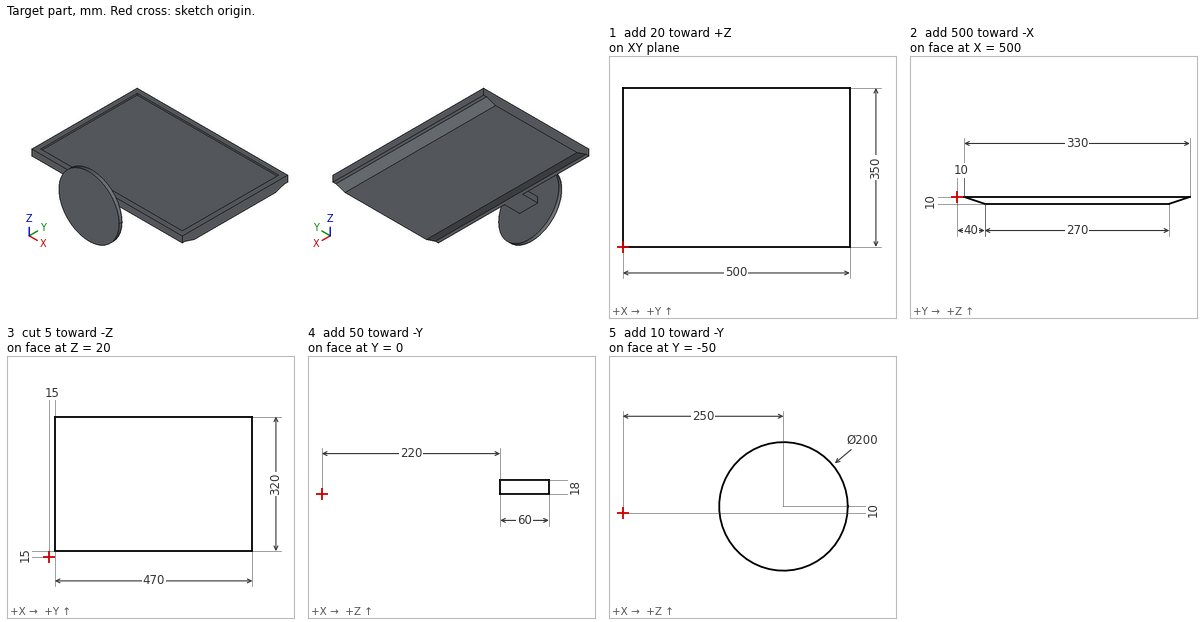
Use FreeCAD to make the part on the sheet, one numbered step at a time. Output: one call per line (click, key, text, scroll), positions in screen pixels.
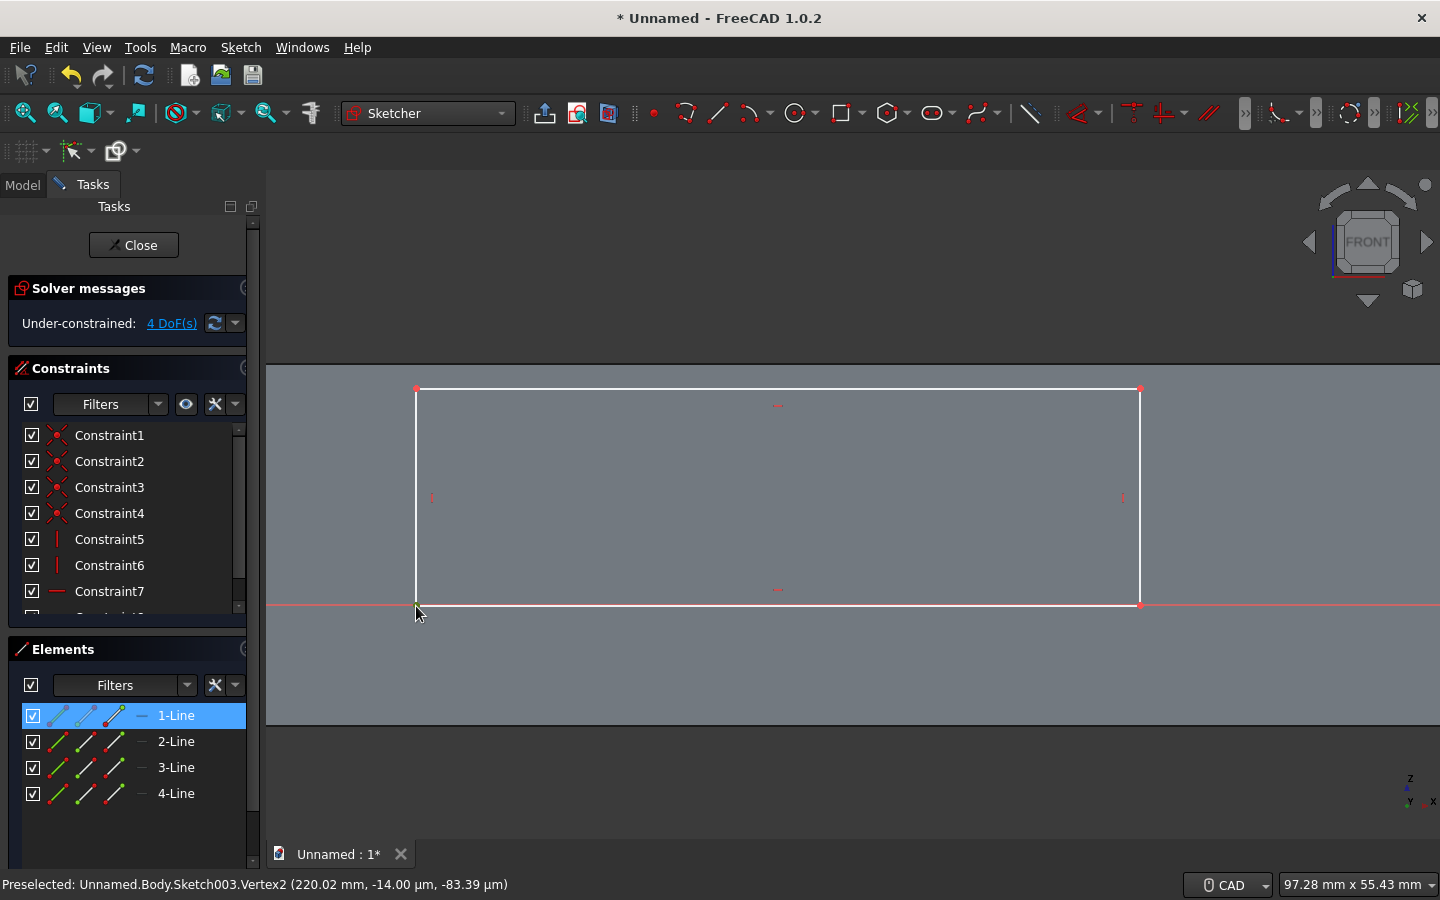
click(364, 605)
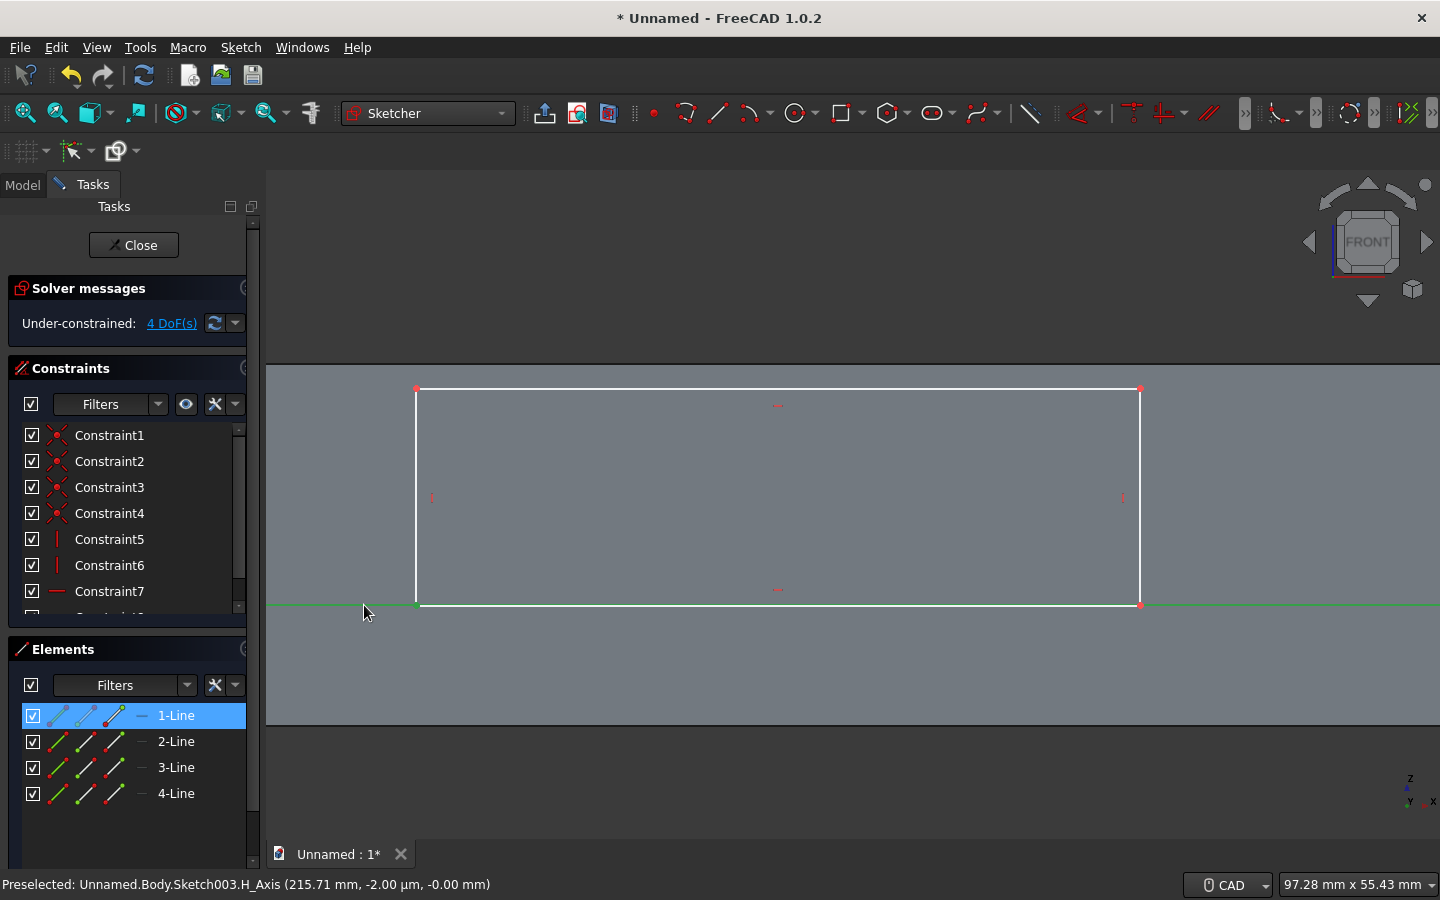
key(c)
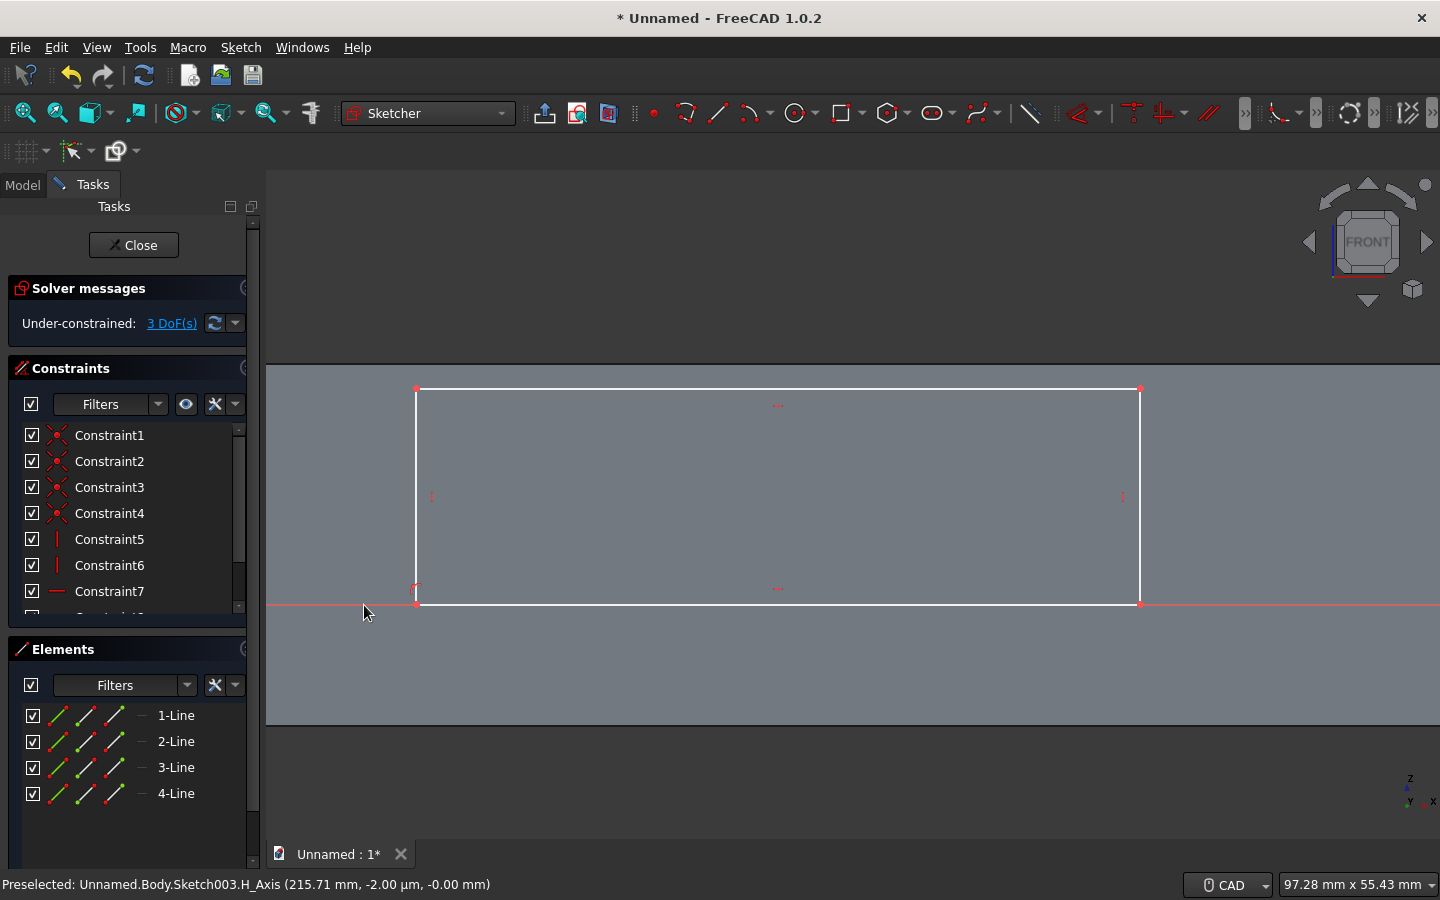
key(d)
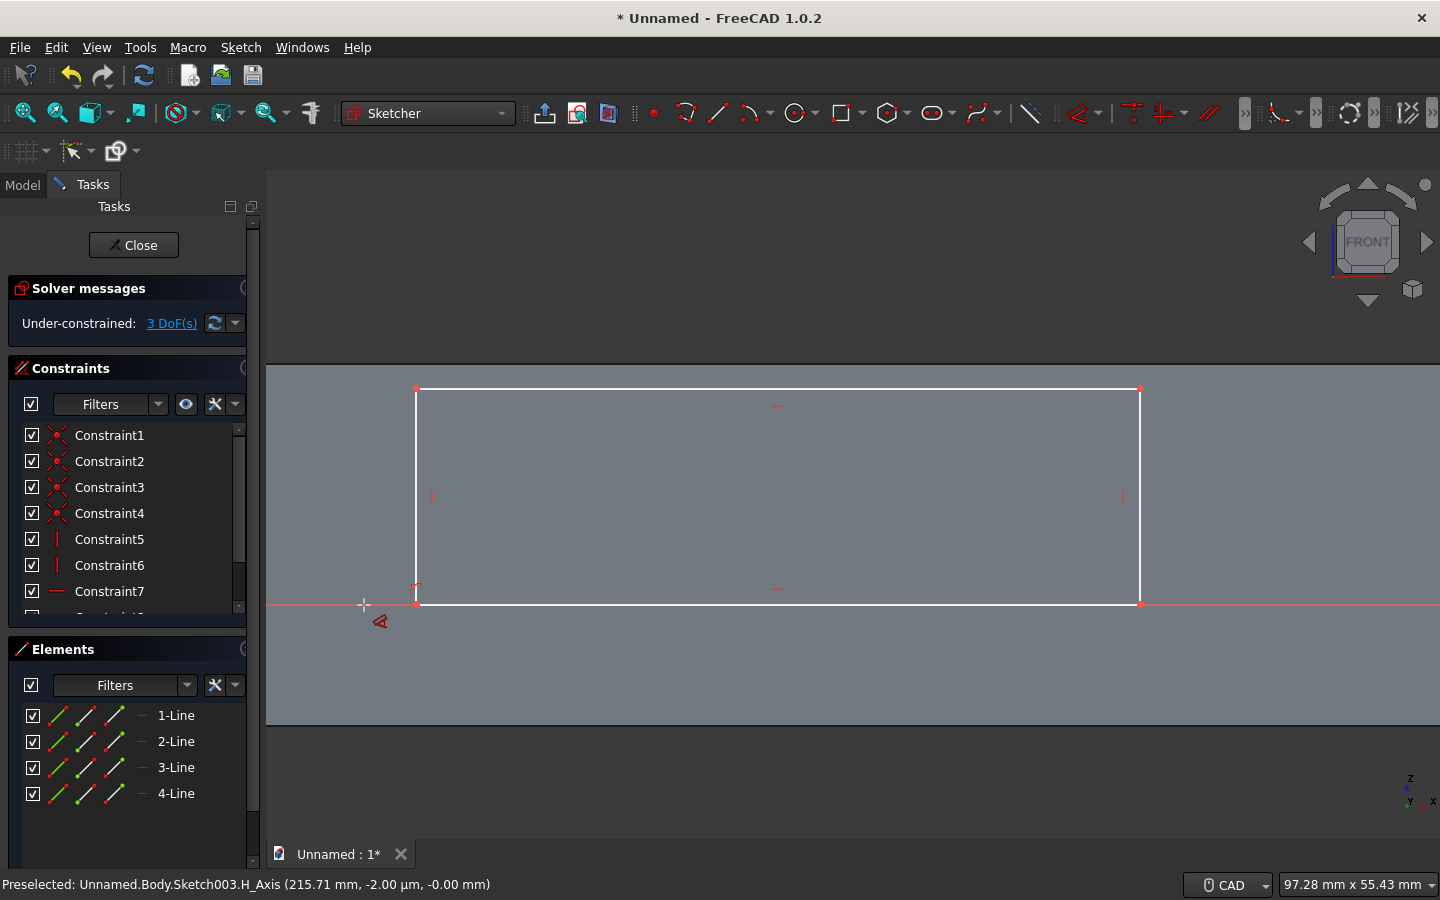
click(416, 454)
click(382, 497)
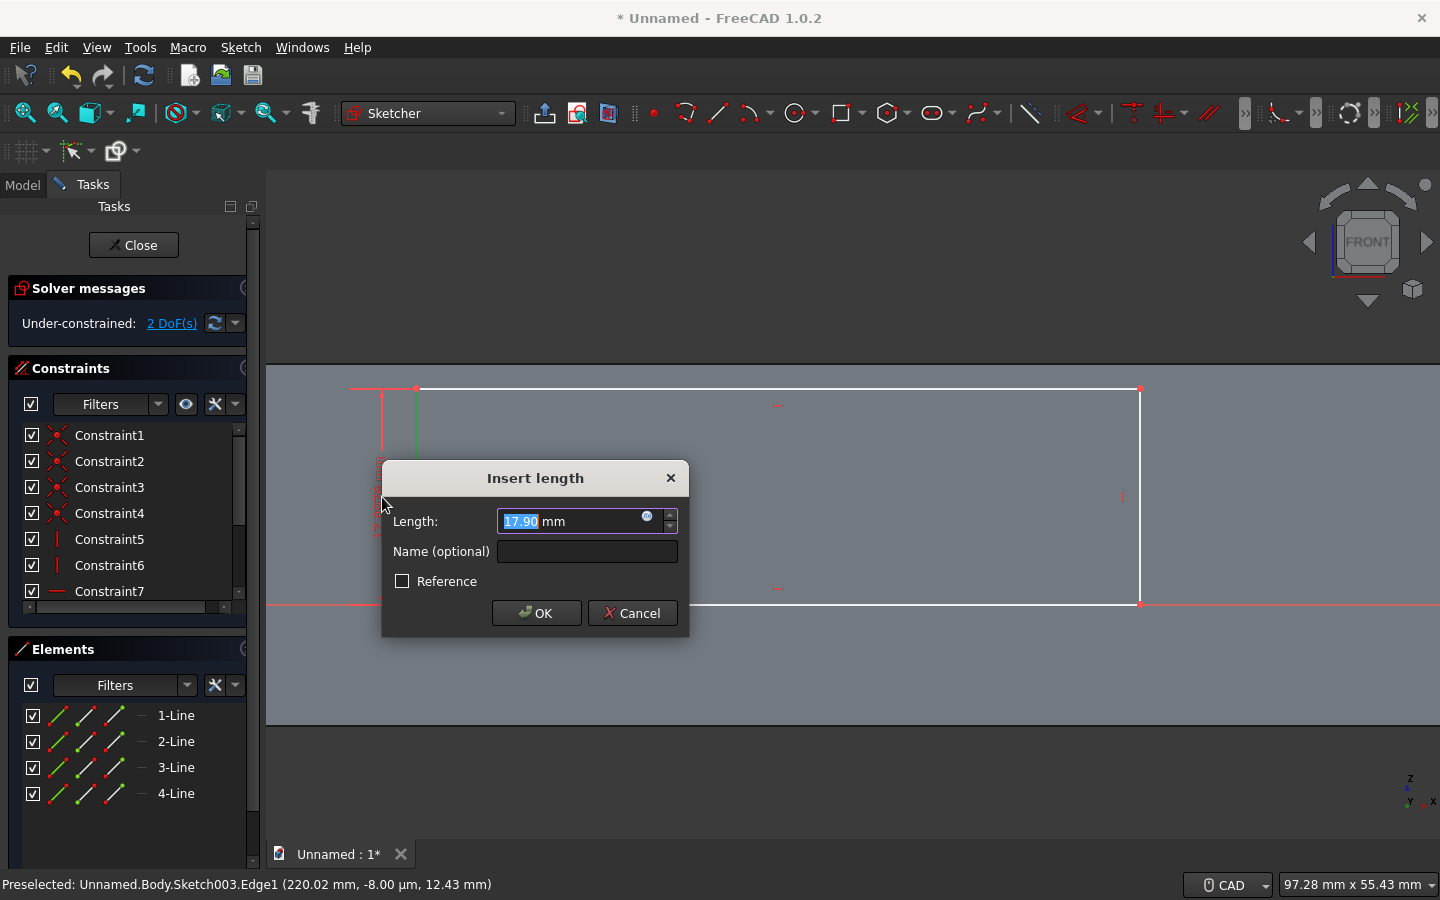
text(18)
key(Return)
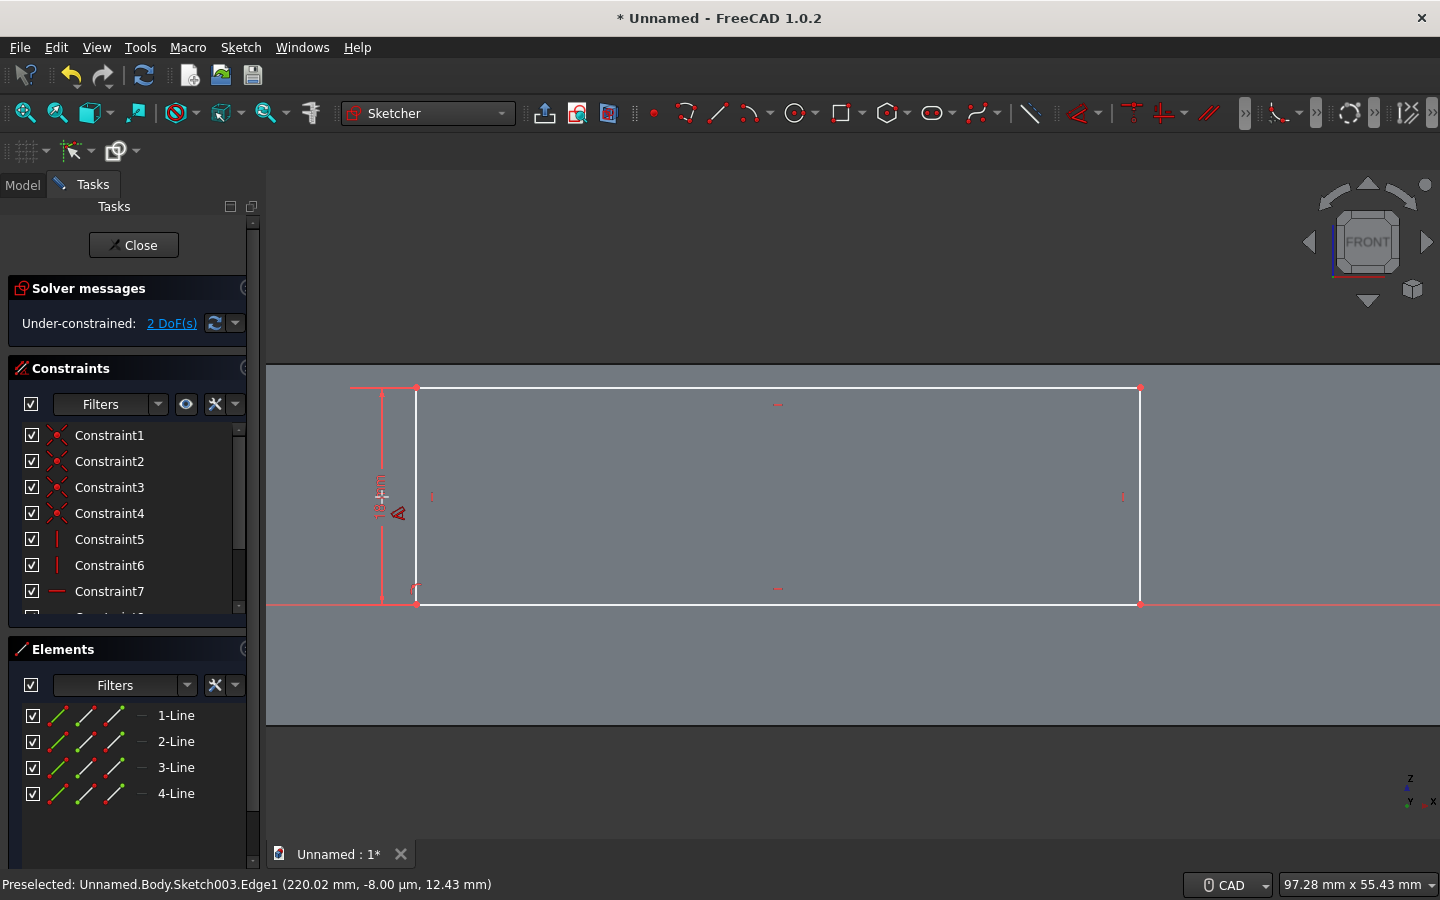
click(633, 605)
click(778, 639)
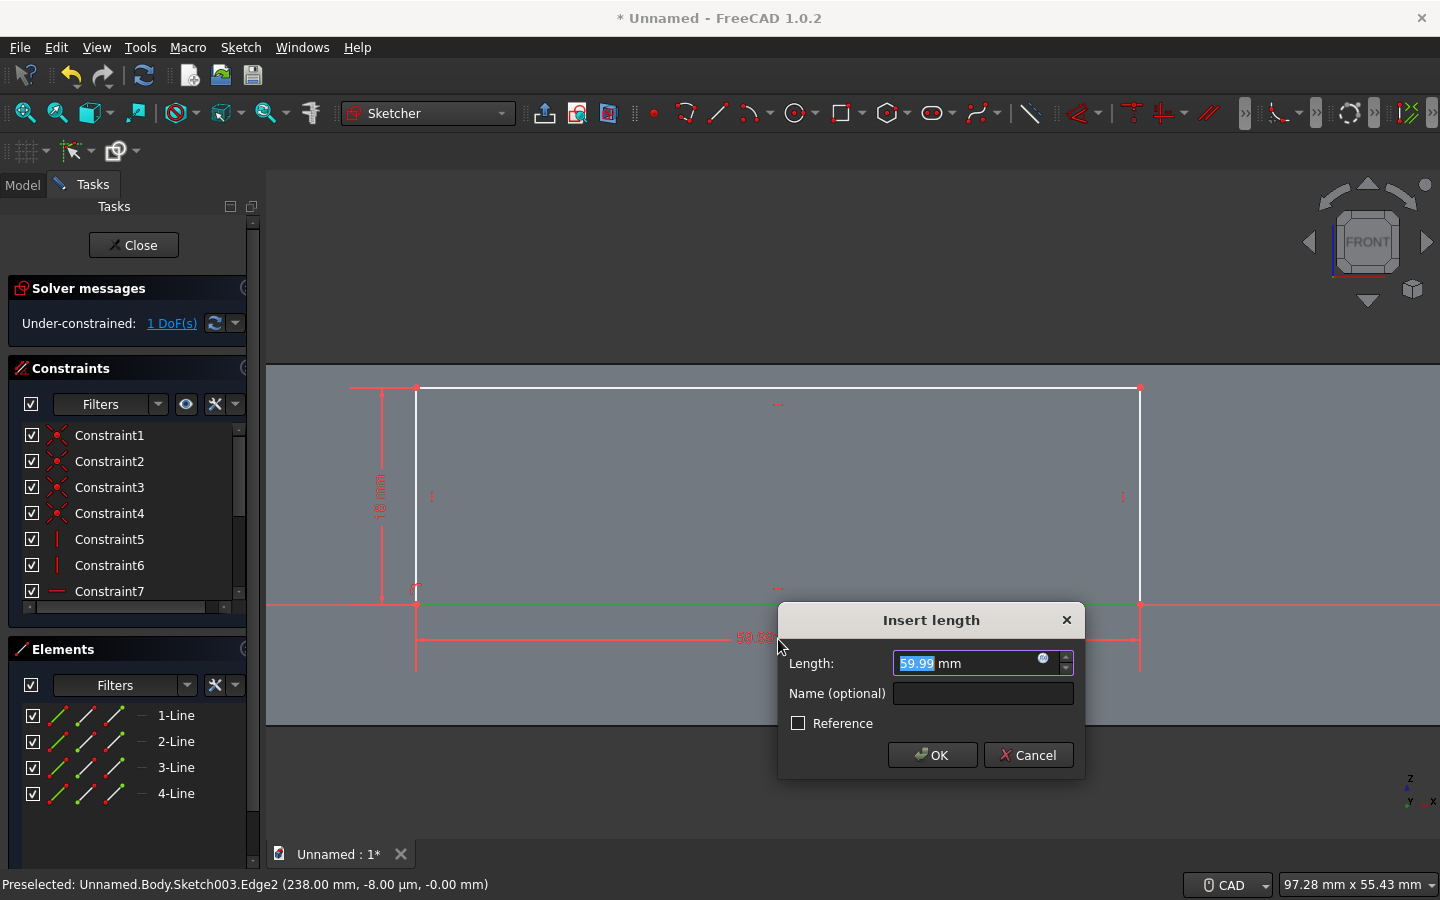
text(60)
key(Return)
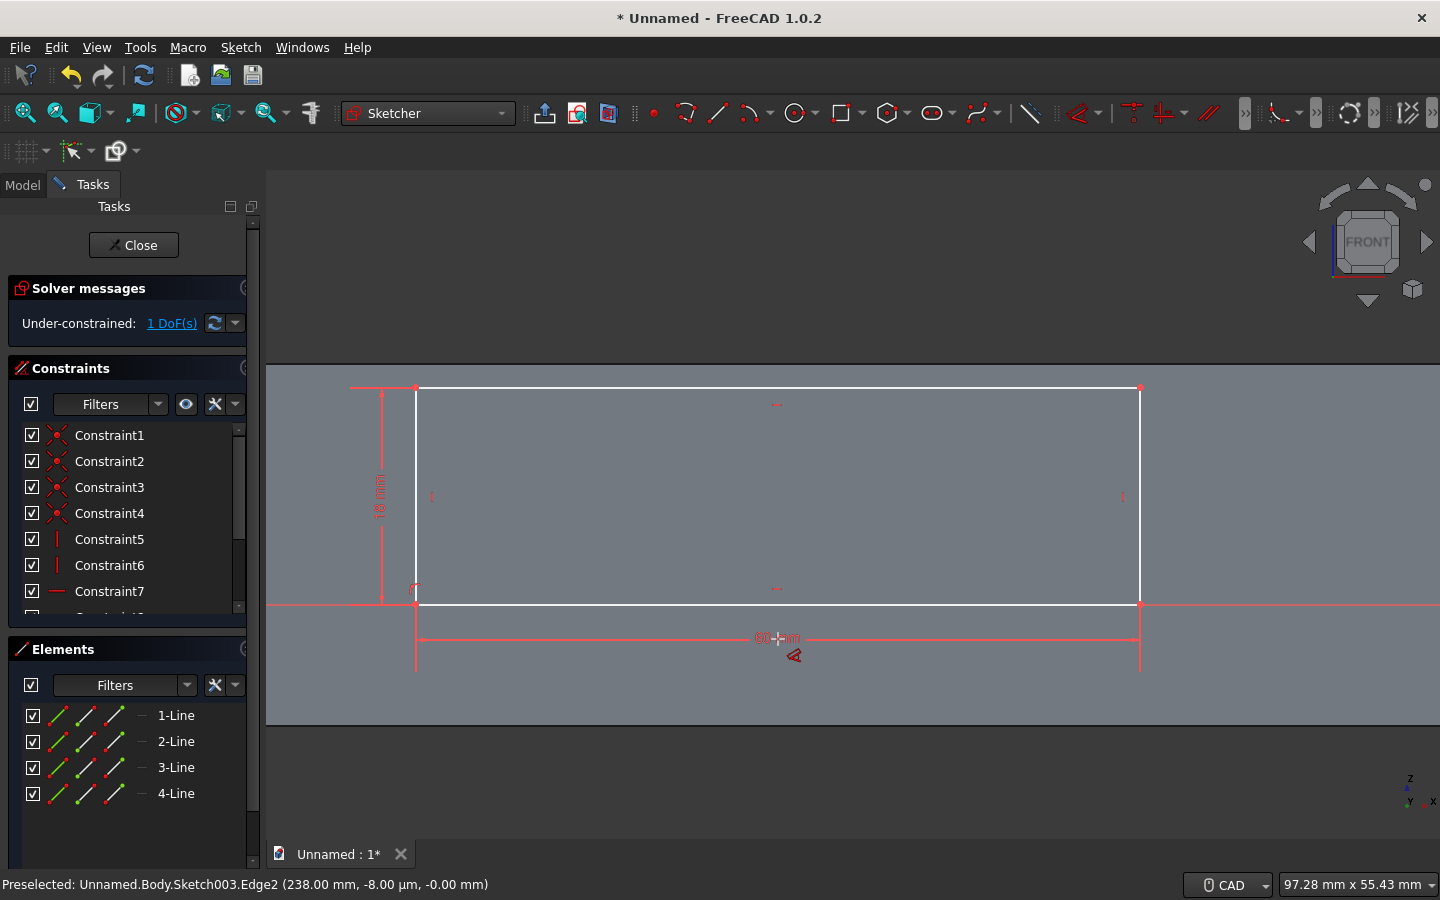
click(416, 388)
click(355, 639)